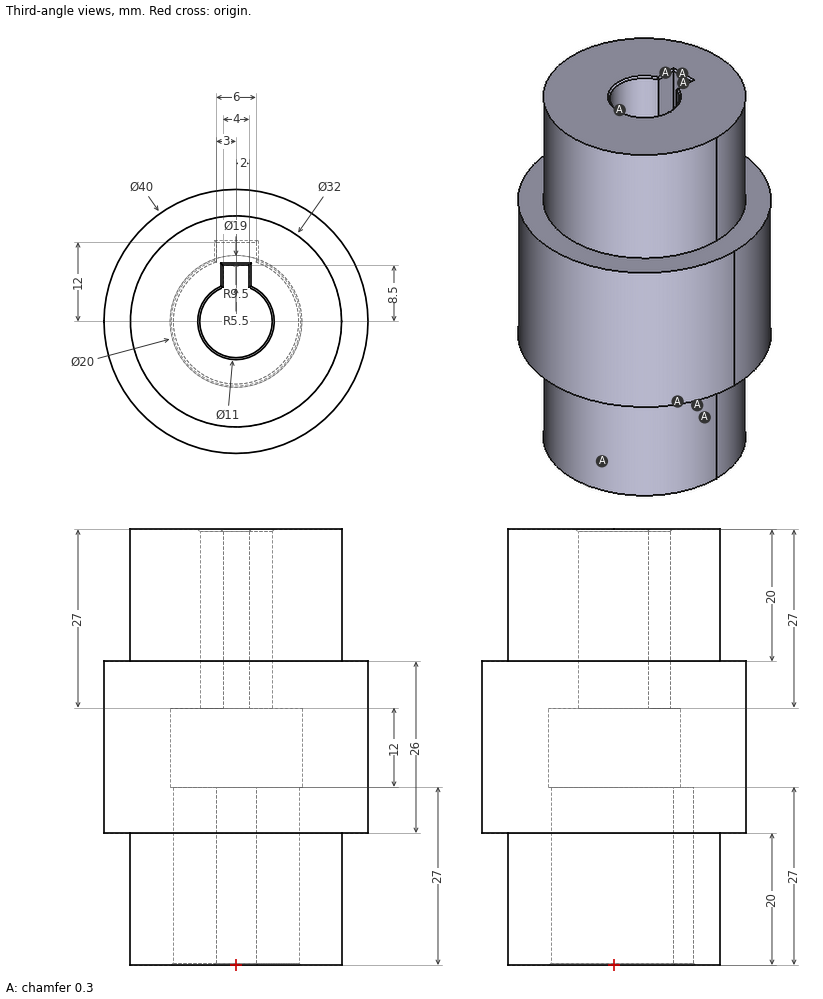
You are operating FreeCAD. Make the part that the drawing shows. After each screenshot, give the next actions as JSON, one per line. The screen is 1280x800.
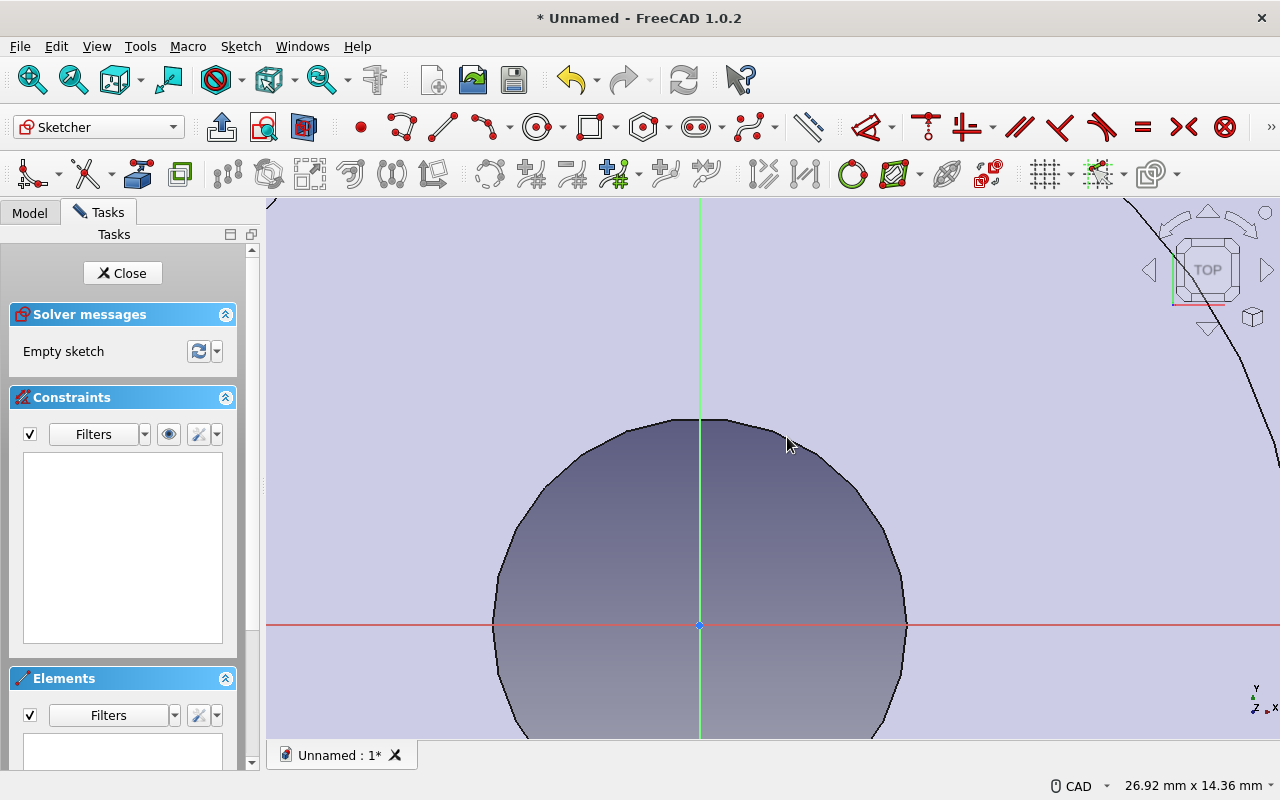
{"action": "left_click", "coordinate": [402, 128]}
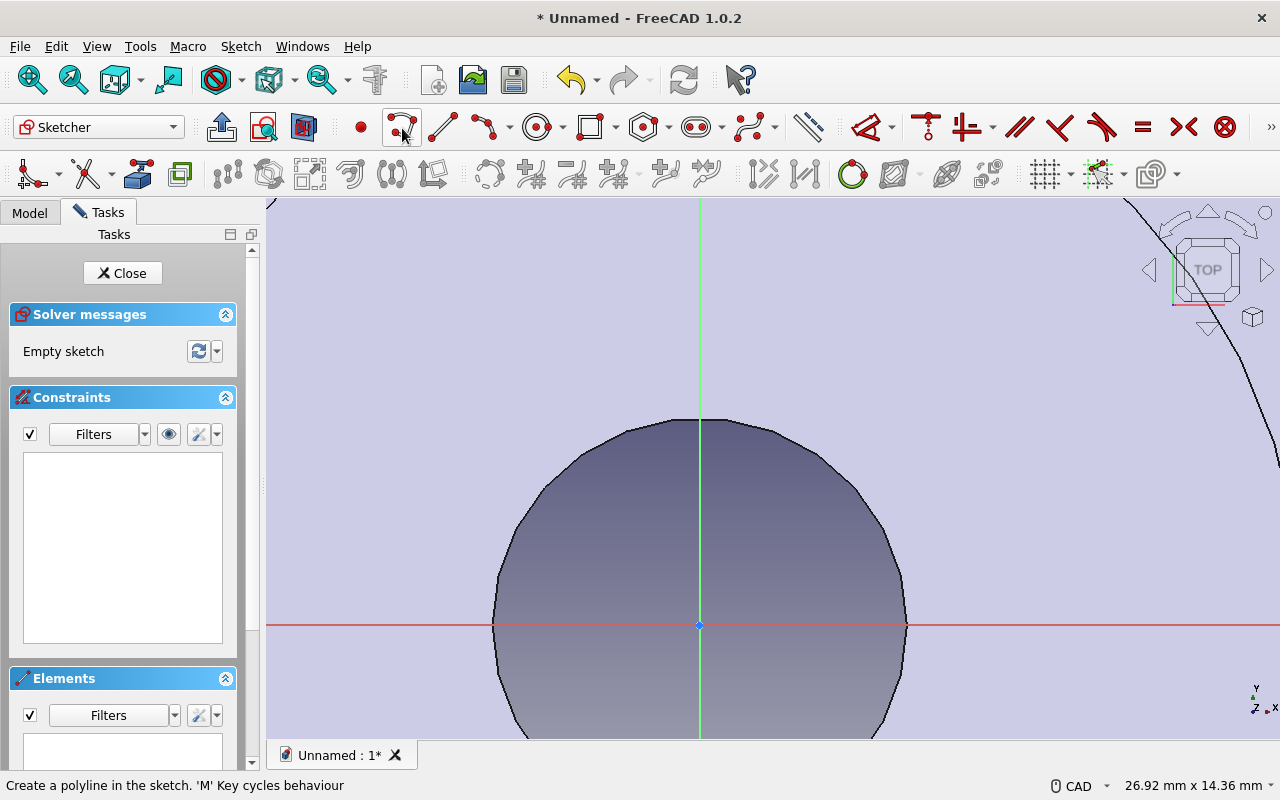
{"action": "left_click", "coordinate": [775, 432]}
{"action": "left_click", "coordinate": [775, 305]}
{"action": "left_click", "coordinate": [624, 305]}
{"action": "left_click", "coordinate": [624, 432]}
{"action": "right_click", "coordinate": [624, 432]}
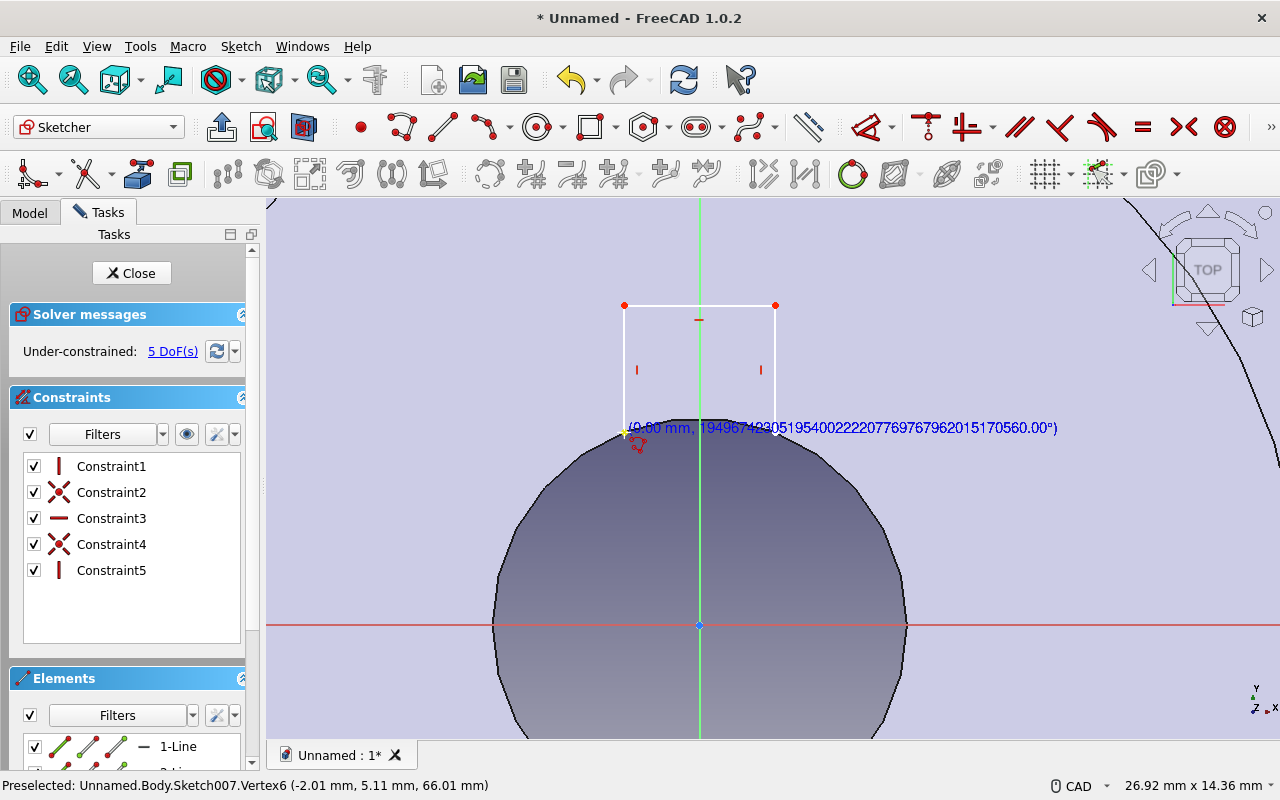
{"action": "left_click", "coordinate": [484, 128]}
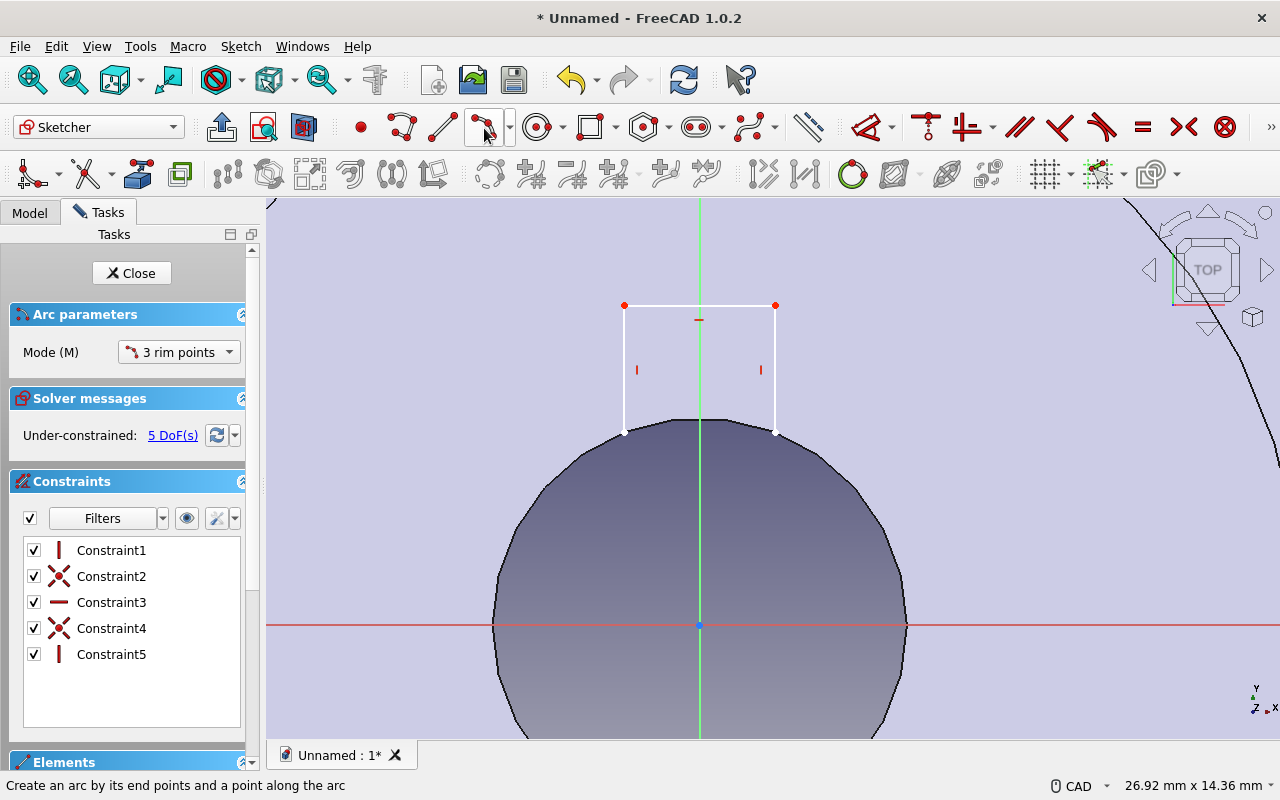
{"action": "left_click", "coordinate": [624, 433]}
{"action": "left_click", "coordinate": [775, 433]}
{"action": "left_click", "coordinate": [715, 419]}
{"action": "key", "text": "Escape"}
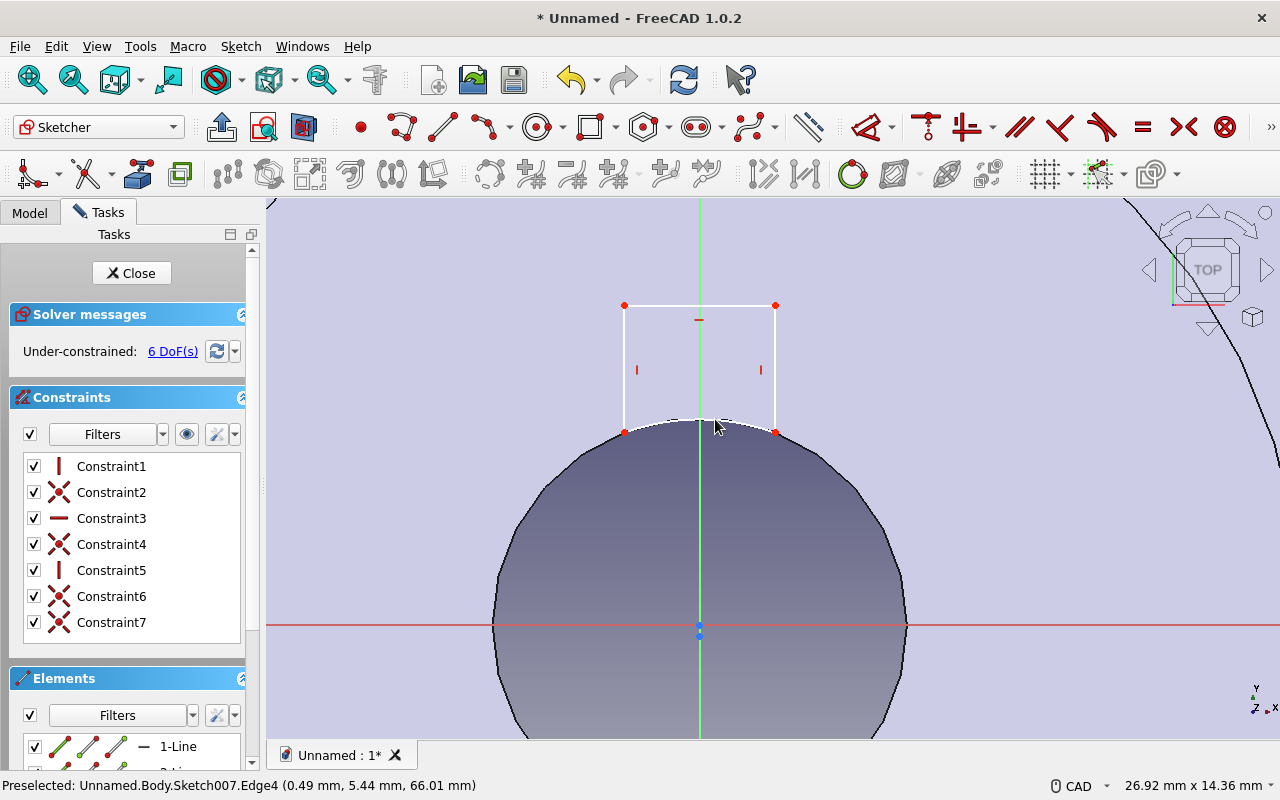
{"action": "left_click_drag", "start_coordinate": [690, 615], "coordinate": [710, 647]}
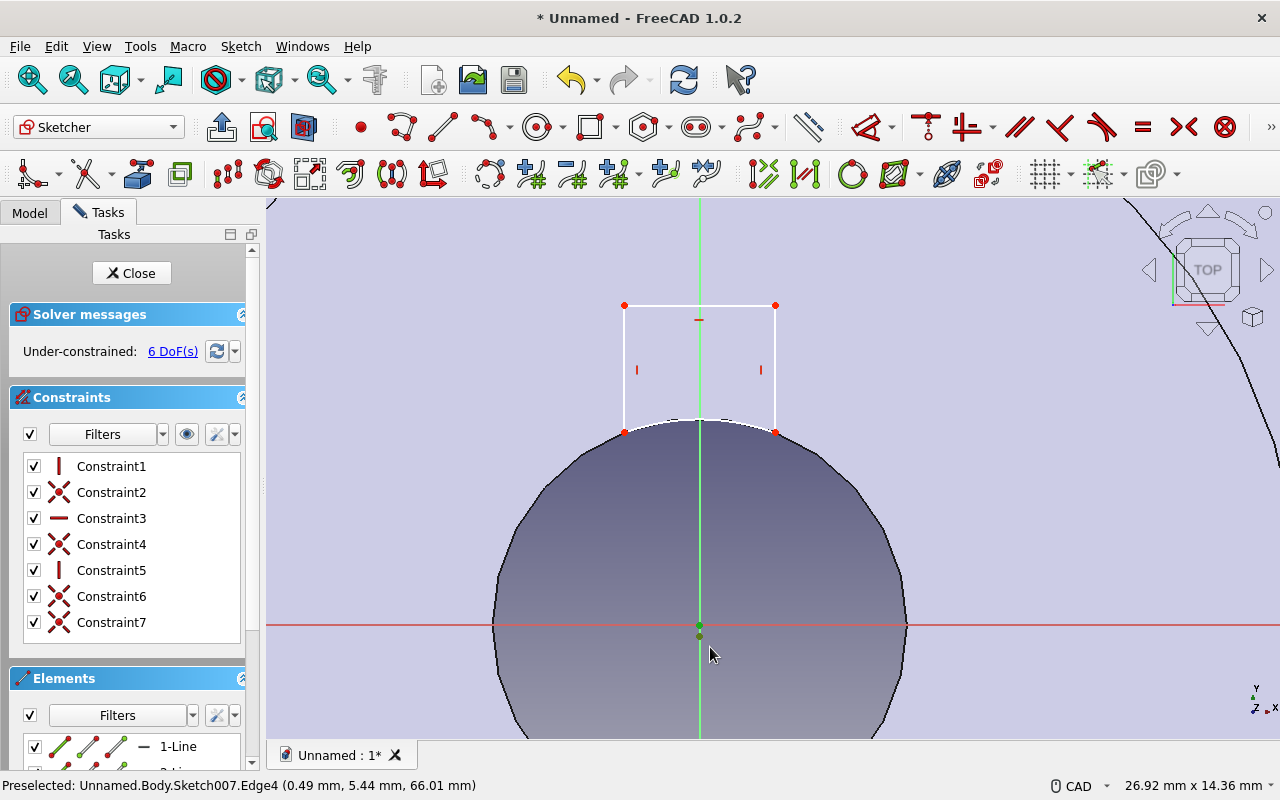
{"action": "left_click", "coordinate": [926, 128]}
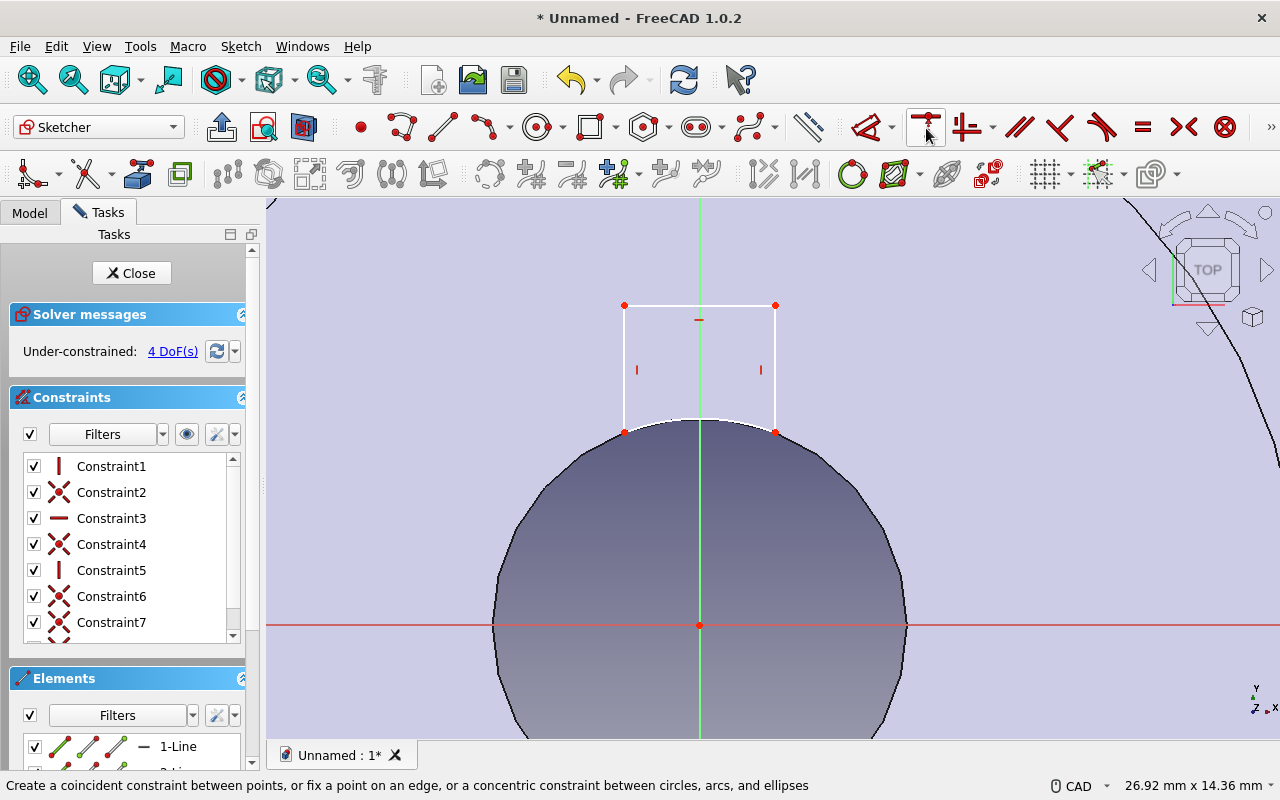
{"action": "left_click", "coordinate": [866, 128]}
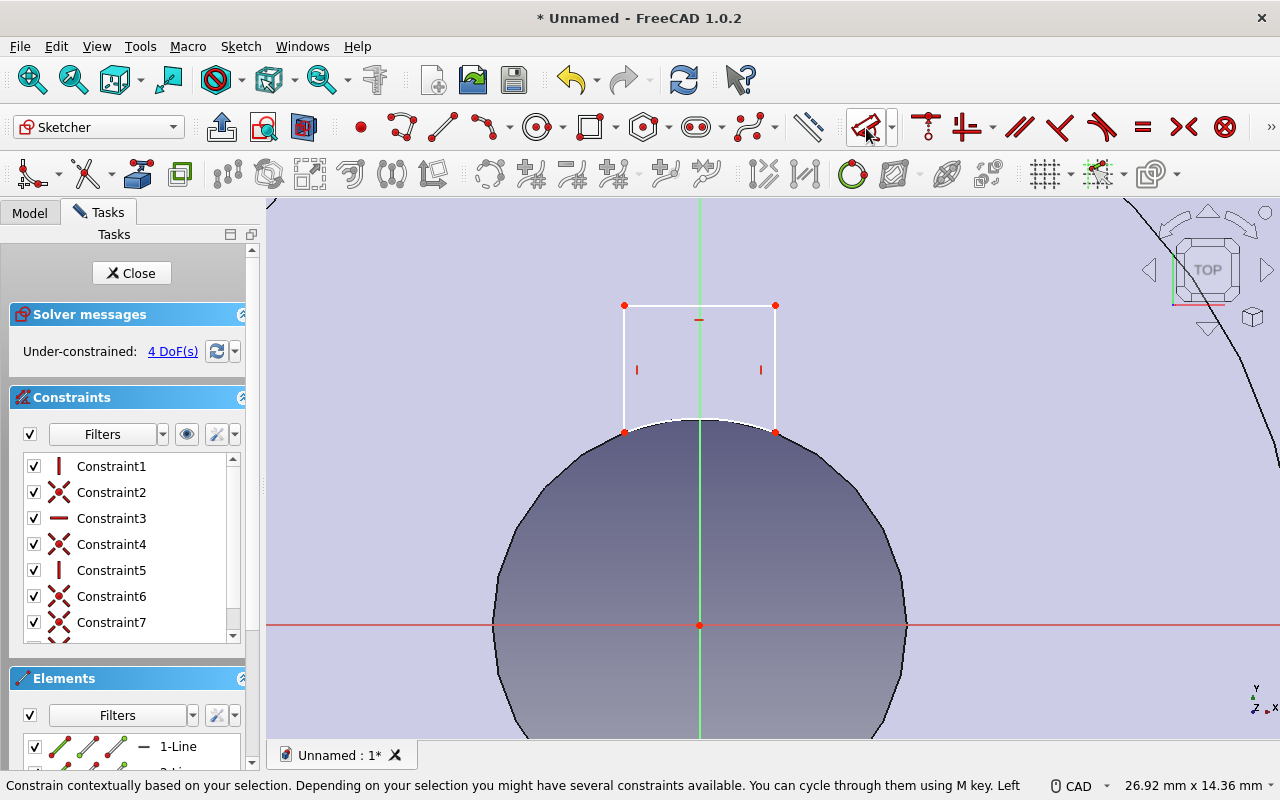
{"action": "left_click", "coordinate": [730, 421]}
{"action": "left_click", "coordinate": [735, 389]}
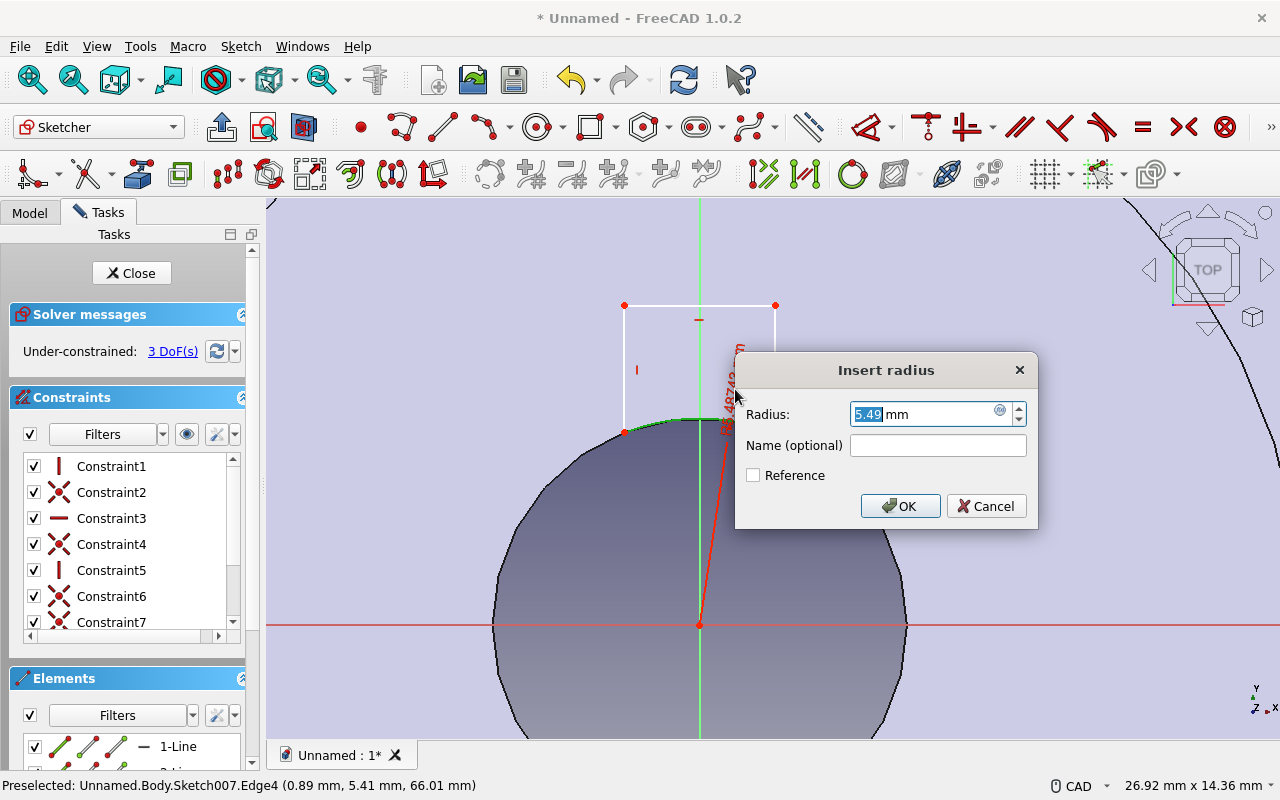
{"action": "type", "text": "5.5"}
{"action": "key", "text": "Return"}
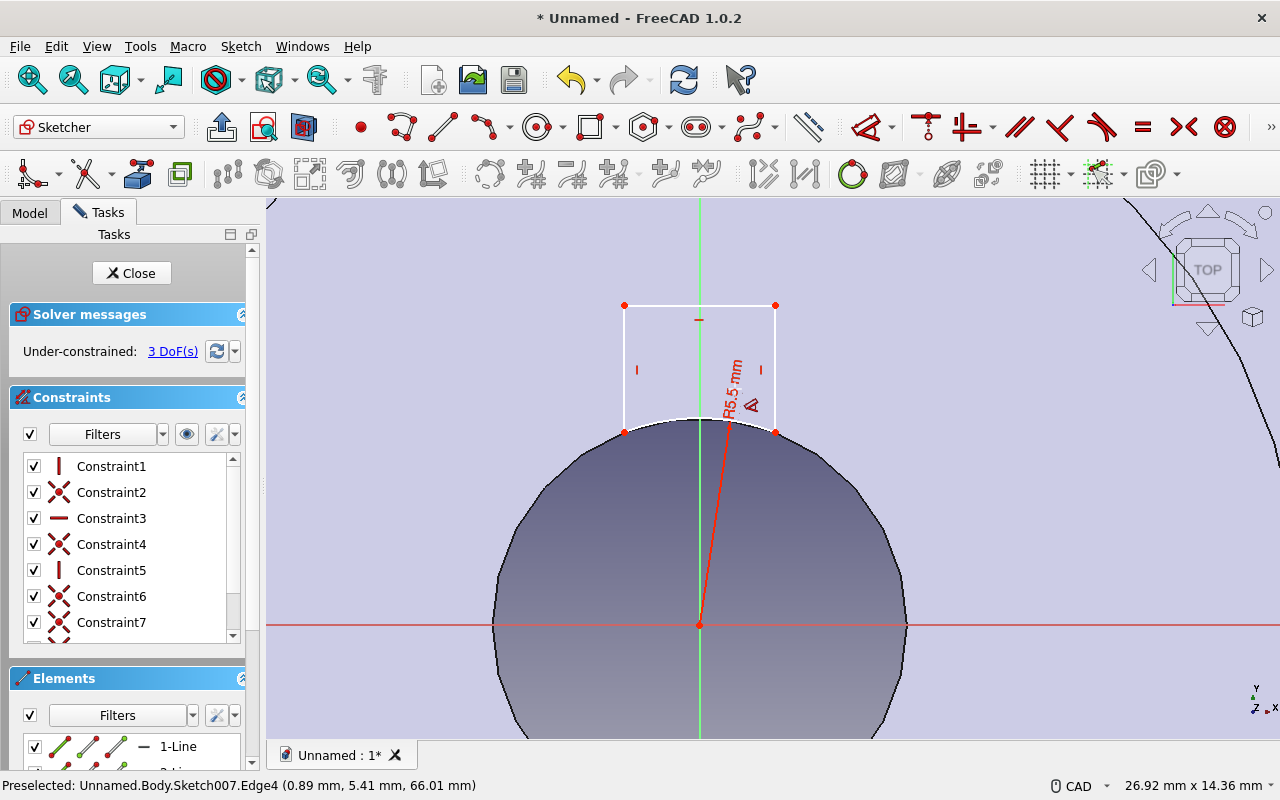
{"action": "left_click", "coordinate": [730, 306]}
{"action": "left_click", "coordinate": [665, 272]}